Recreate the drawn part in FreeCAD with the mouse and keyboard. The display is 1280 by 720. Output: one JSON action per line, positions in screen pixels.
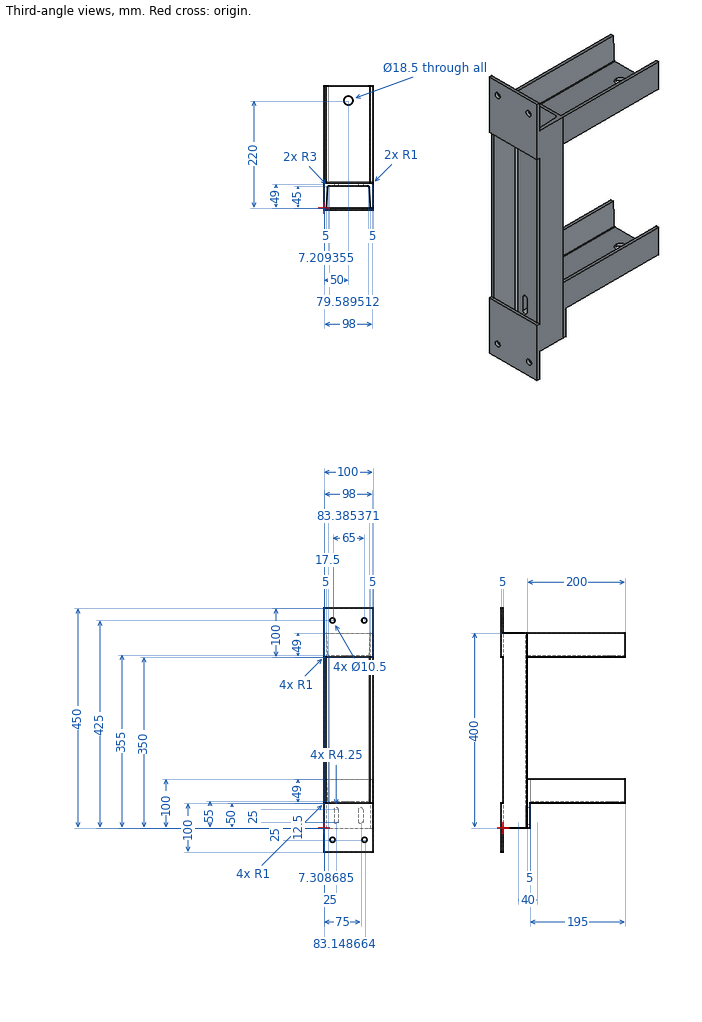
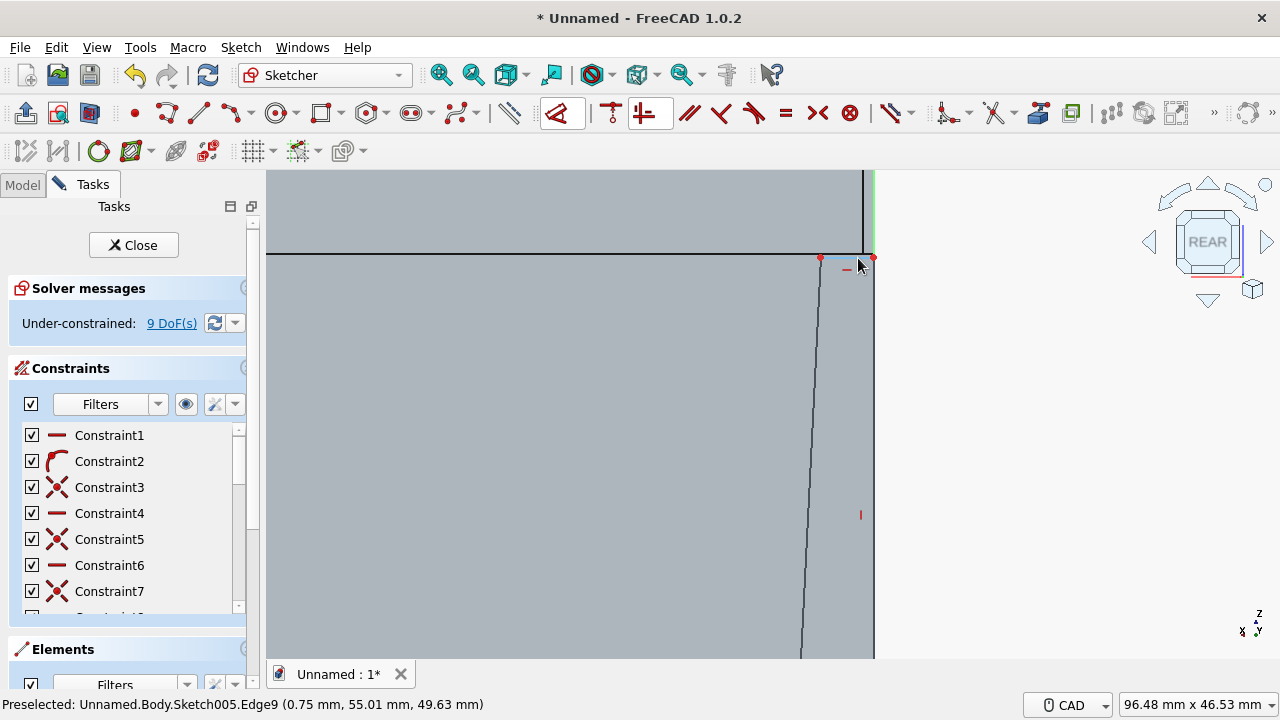
{"action": "left_click", "coordinate": [858, 258]}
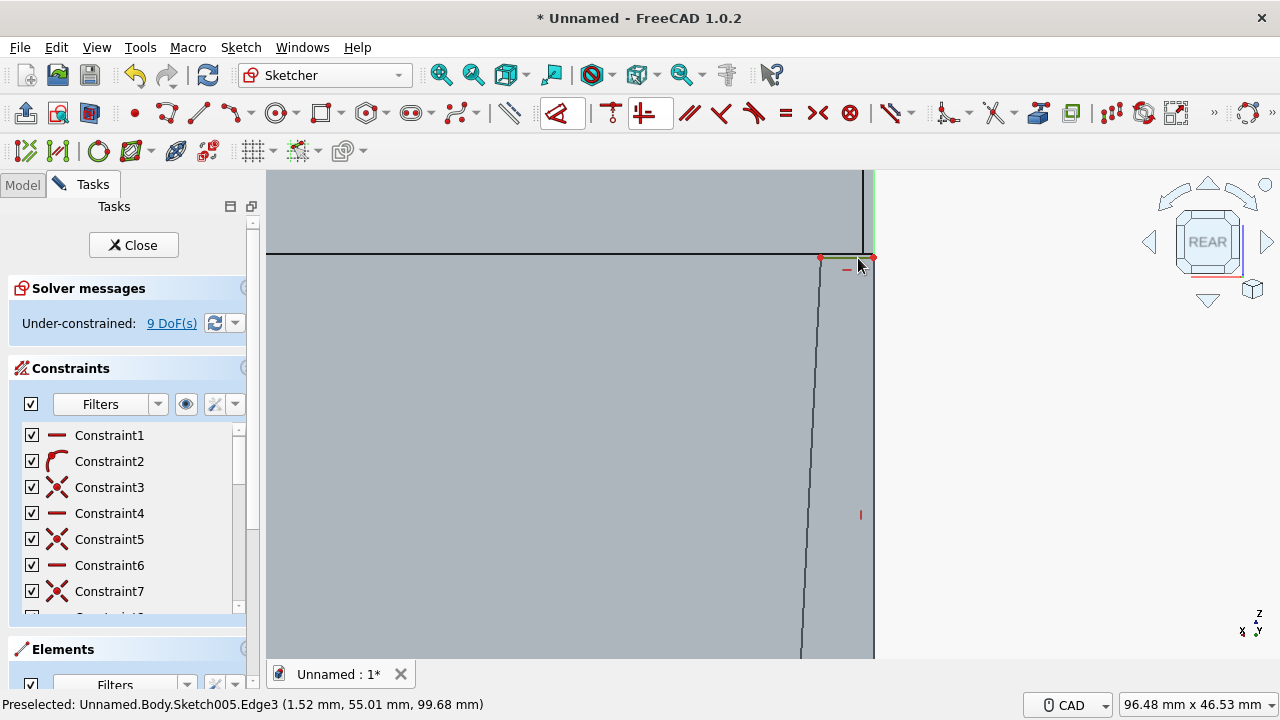
{"action": "key", "text": "l"}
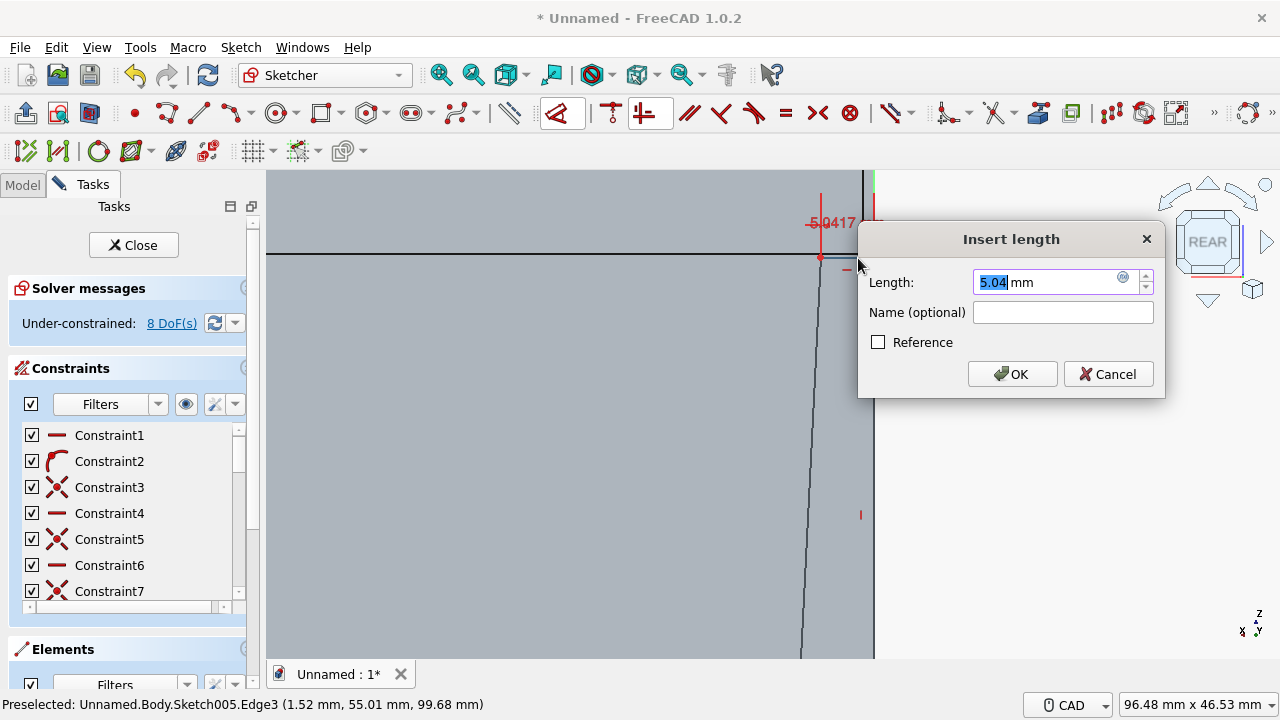
{"action": "type", "text": "5"}
{"action": "key", "text": "Return"}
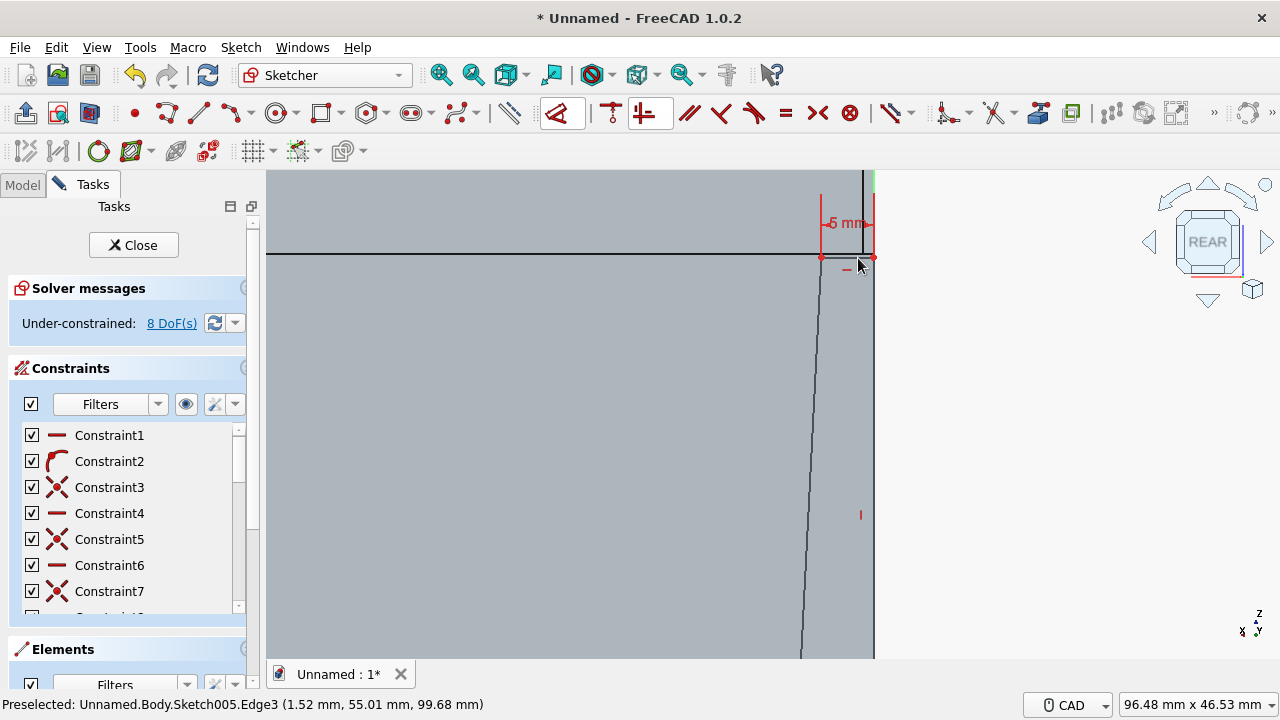
{"action": "scroll", "coordinate": [858, 257], "scroll_direction": "down", "scroll_amount": 6}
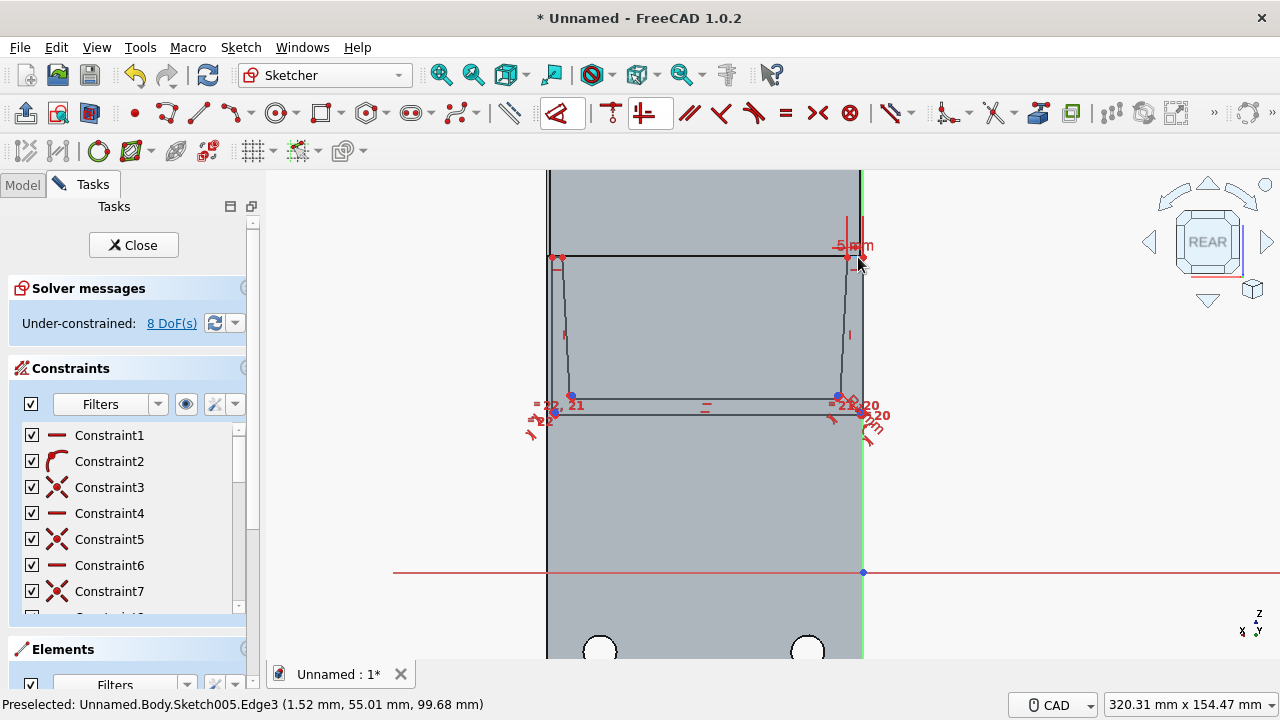
{"action": "scroll", "coordinate": [559, 257], "scroll_direction": "up", "scroll_amount": 8}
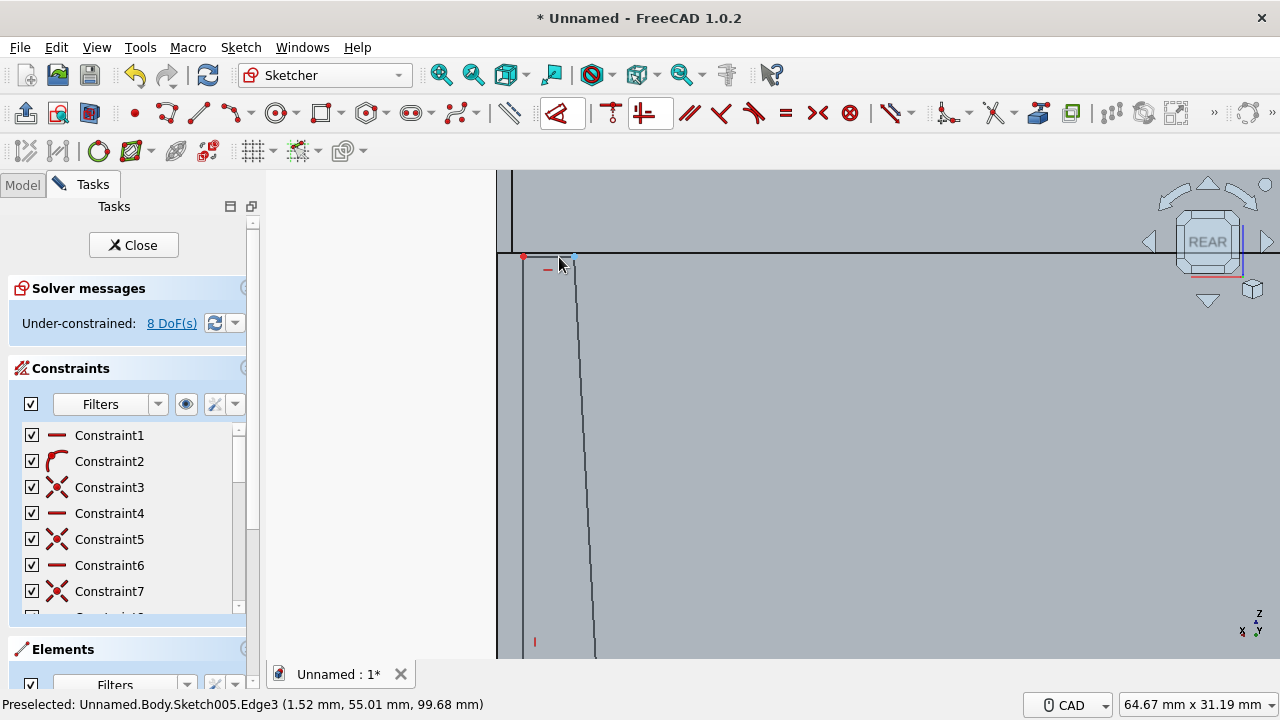
{"action": "left_click", "coordinate": [559, 257]}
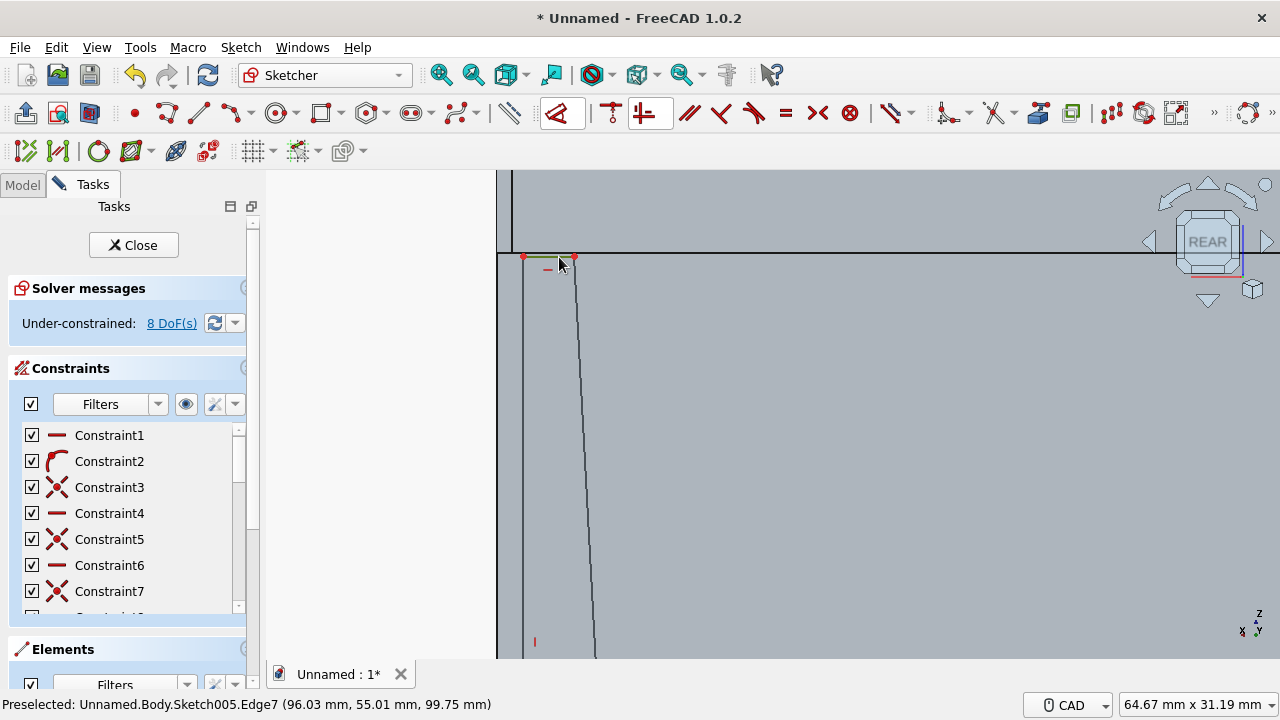
{"action": "key", "text": "l"}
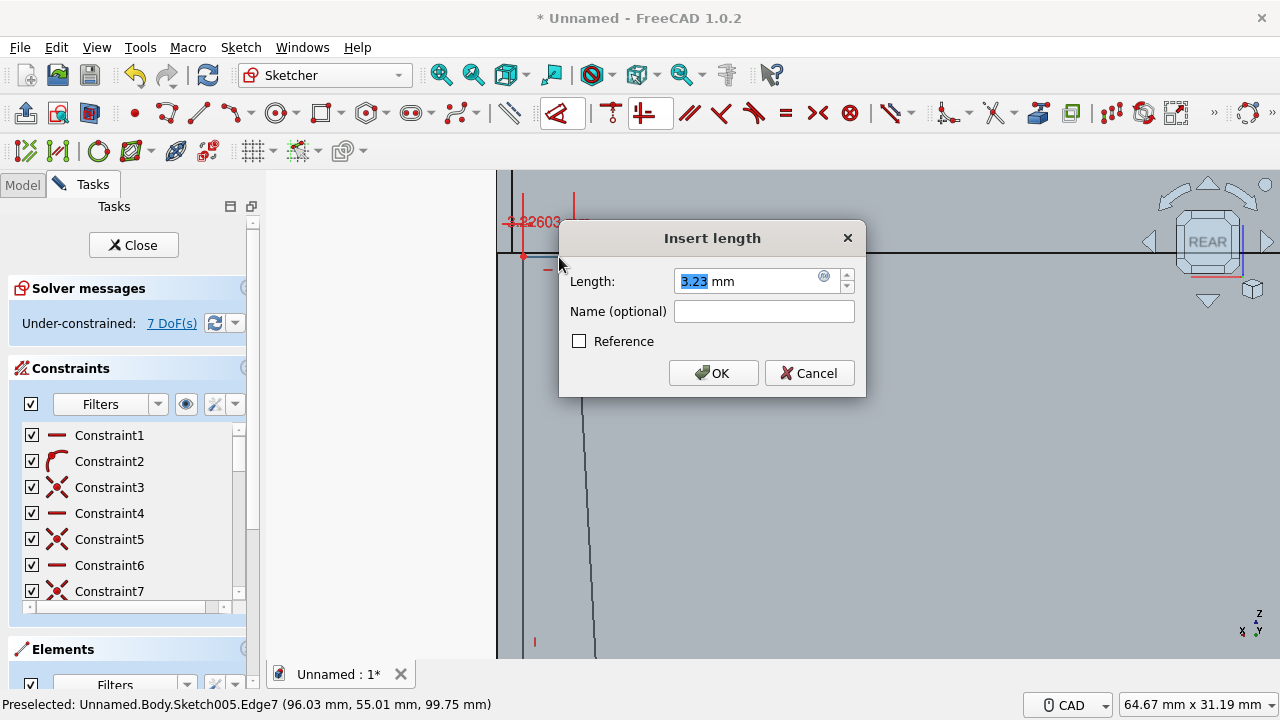
{"action": "type", "text": "5"}
{"action": "key", "text": "Return"}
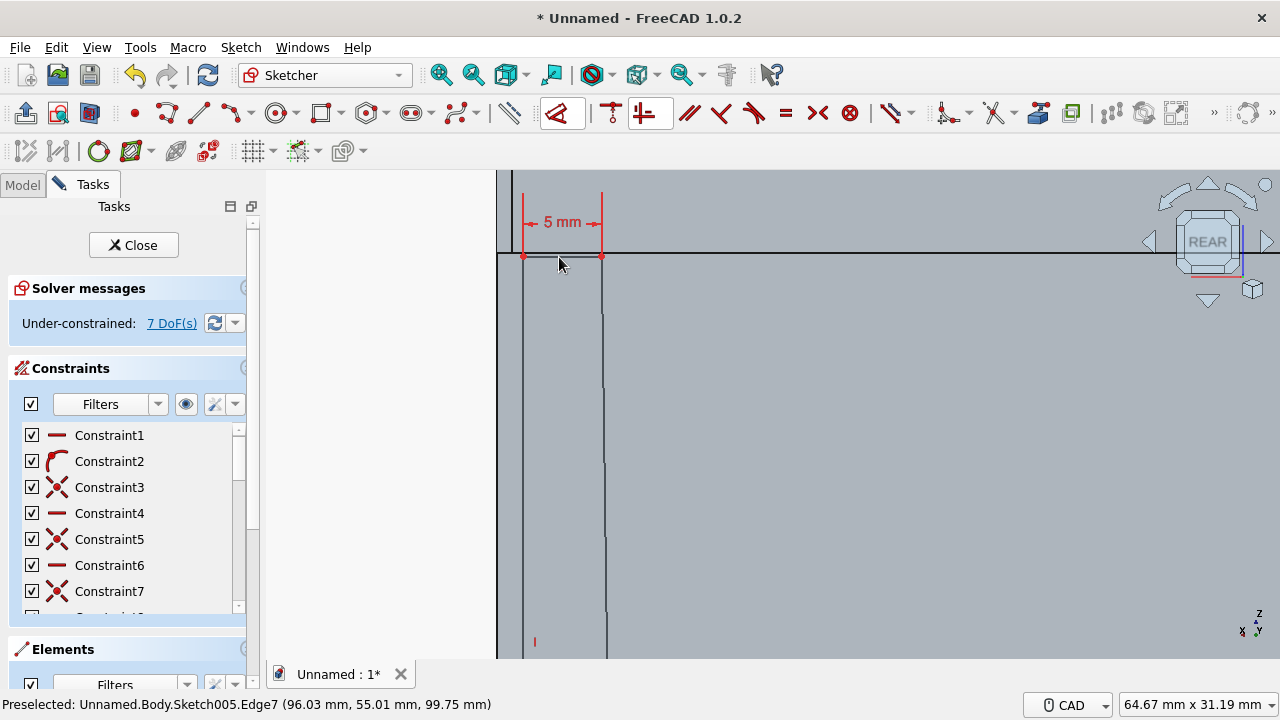
{"action": "scroll", "coordinate": [559, 257], "scroll_direction": "down", "scroll_amount": 8}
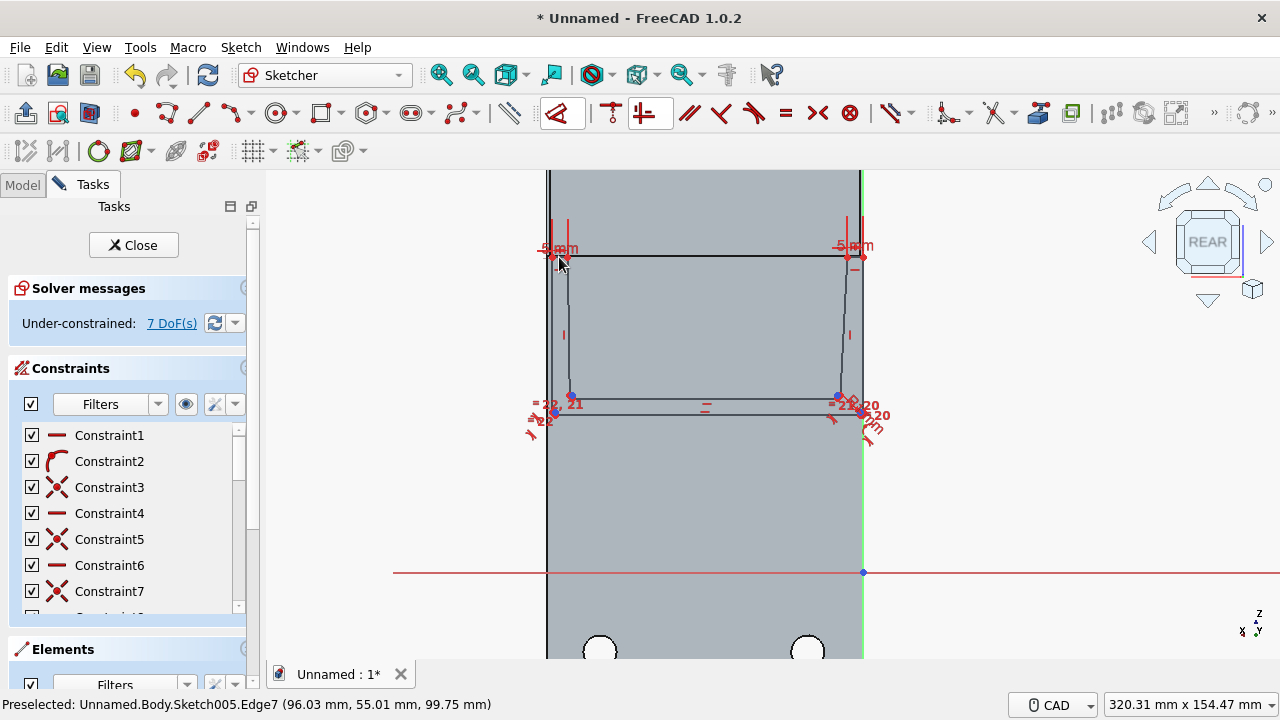
{"action": "left_click", "coordinate": [647, 415]}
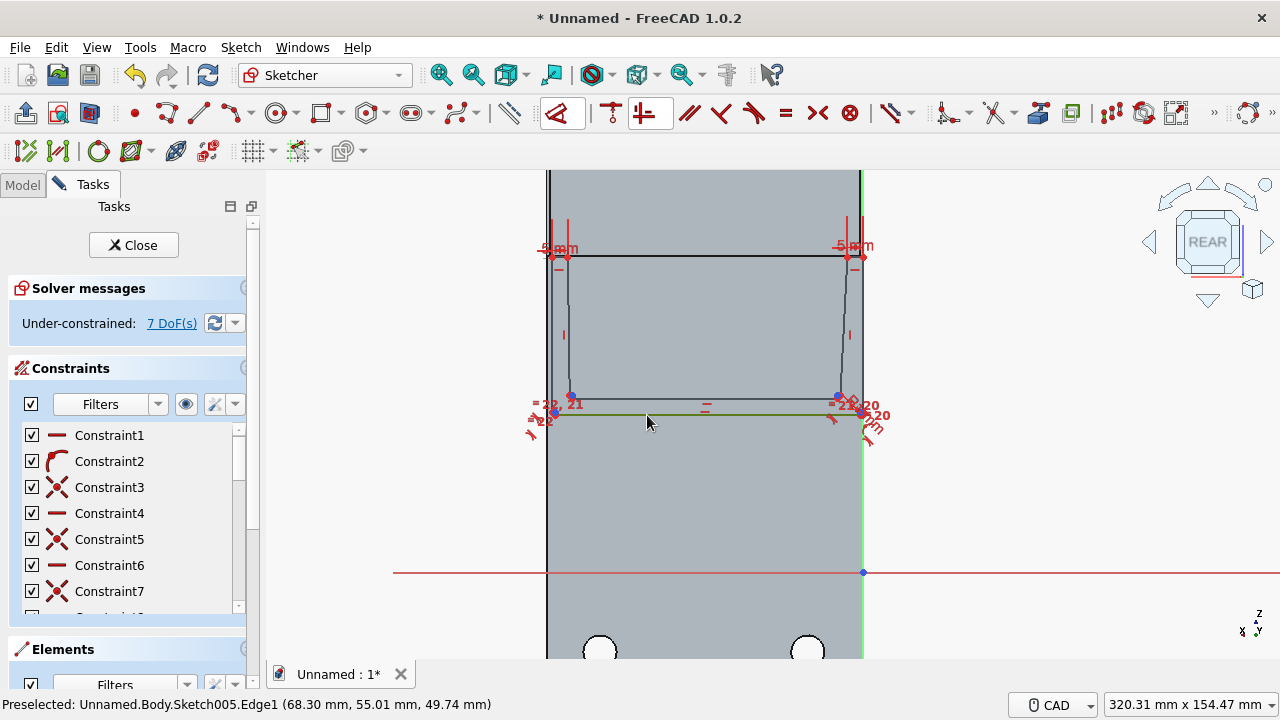
{"action": "left_click", "coordinate": [580, 114]}